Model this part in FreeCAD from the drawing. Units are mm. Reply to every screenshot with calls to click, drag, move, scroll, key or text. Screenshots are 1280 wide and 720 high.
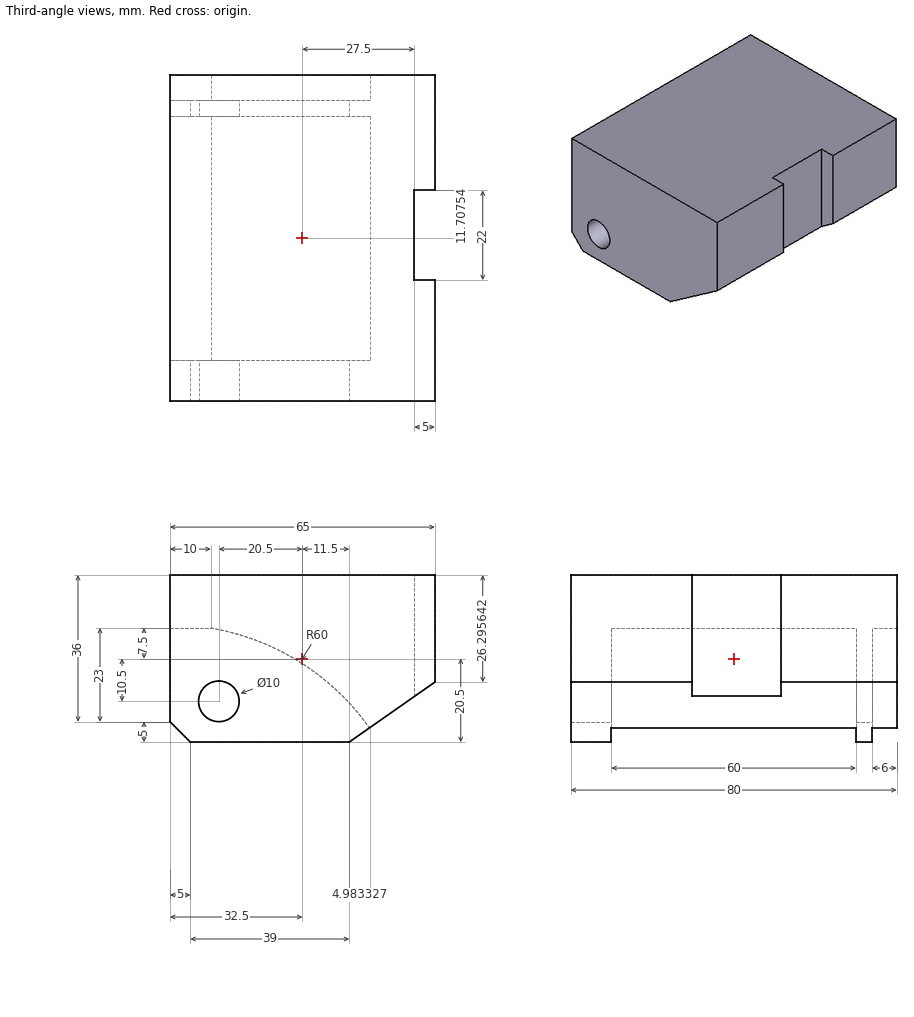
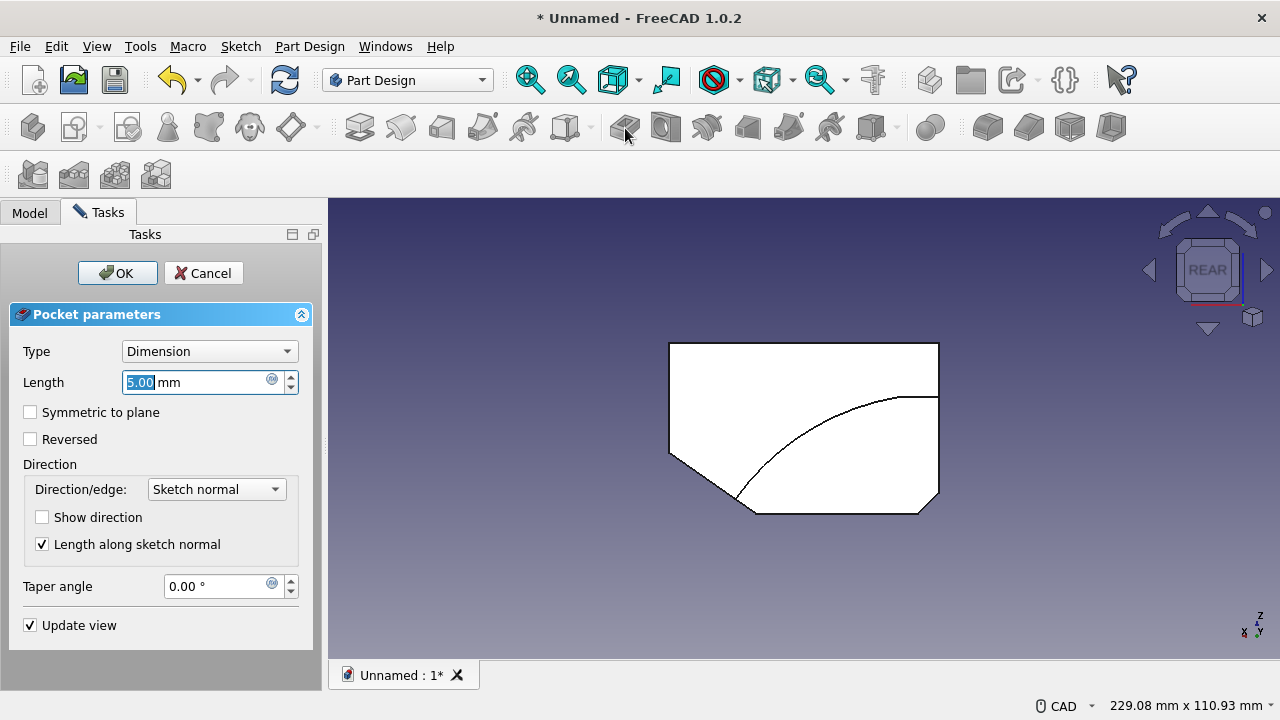
text(60)
key(Tab)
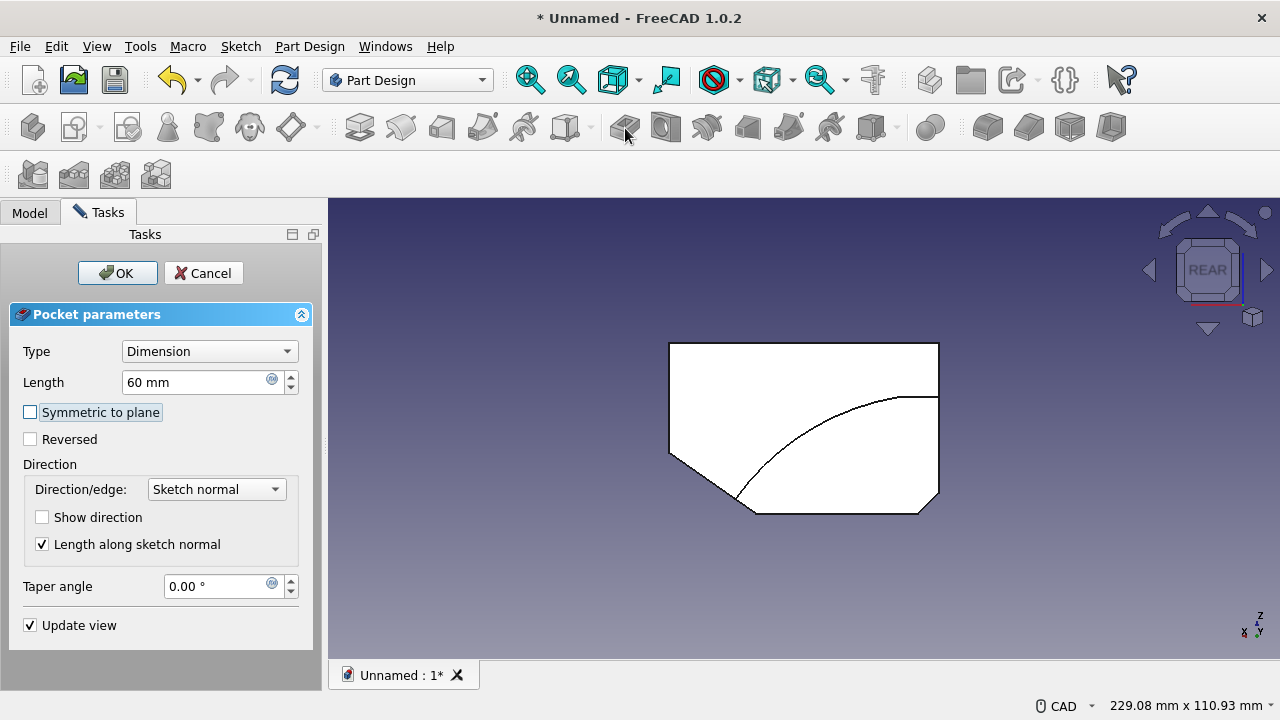
click(31, 412)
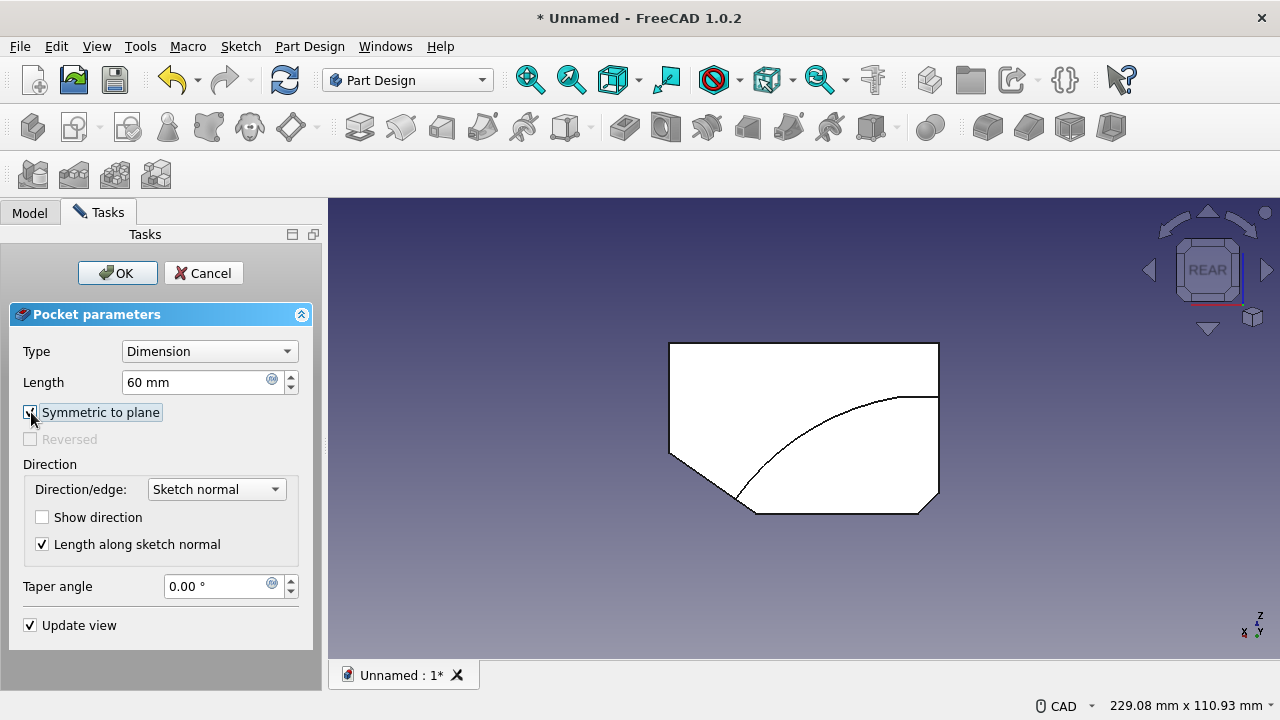
click(118, 273)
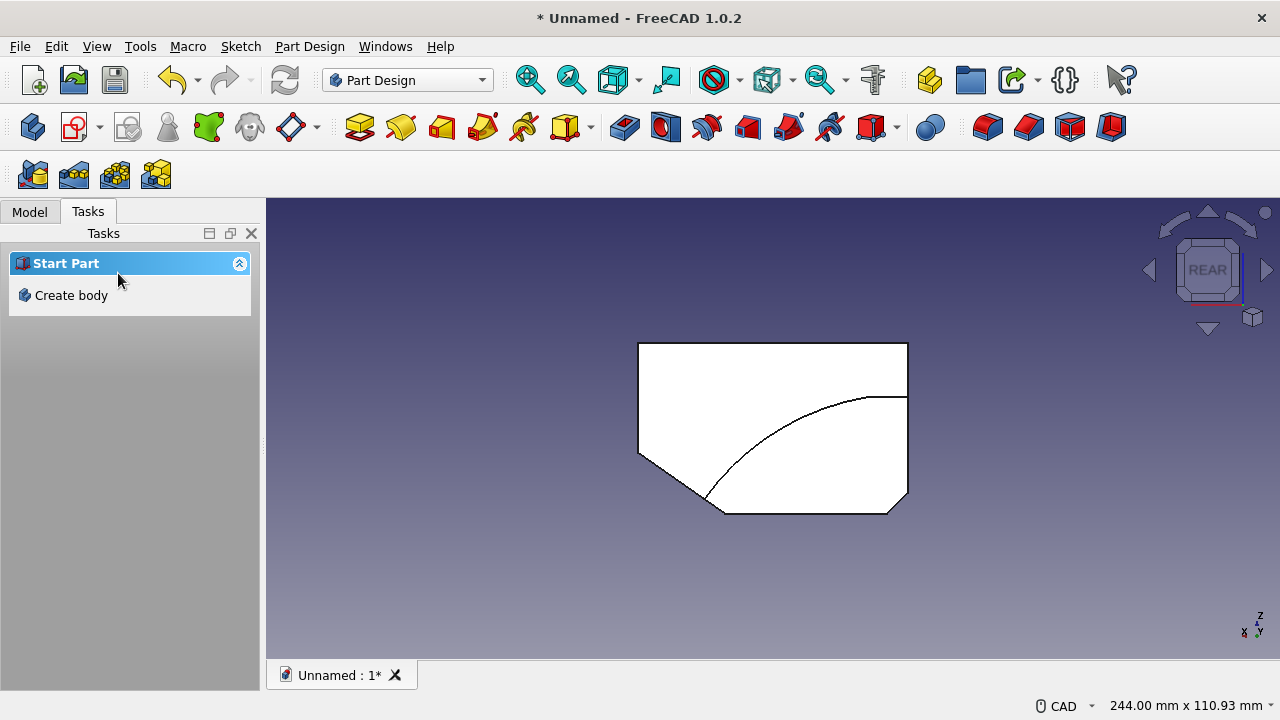
key(v)
key(f)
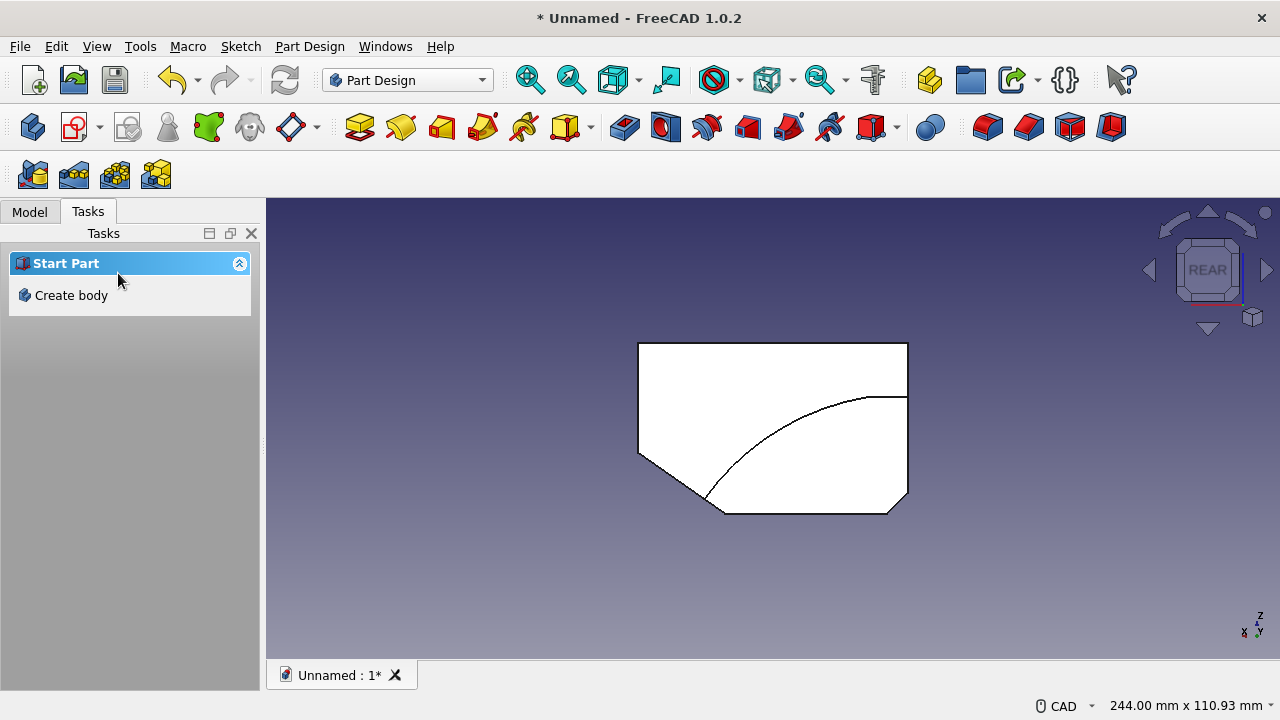
click(835, 455)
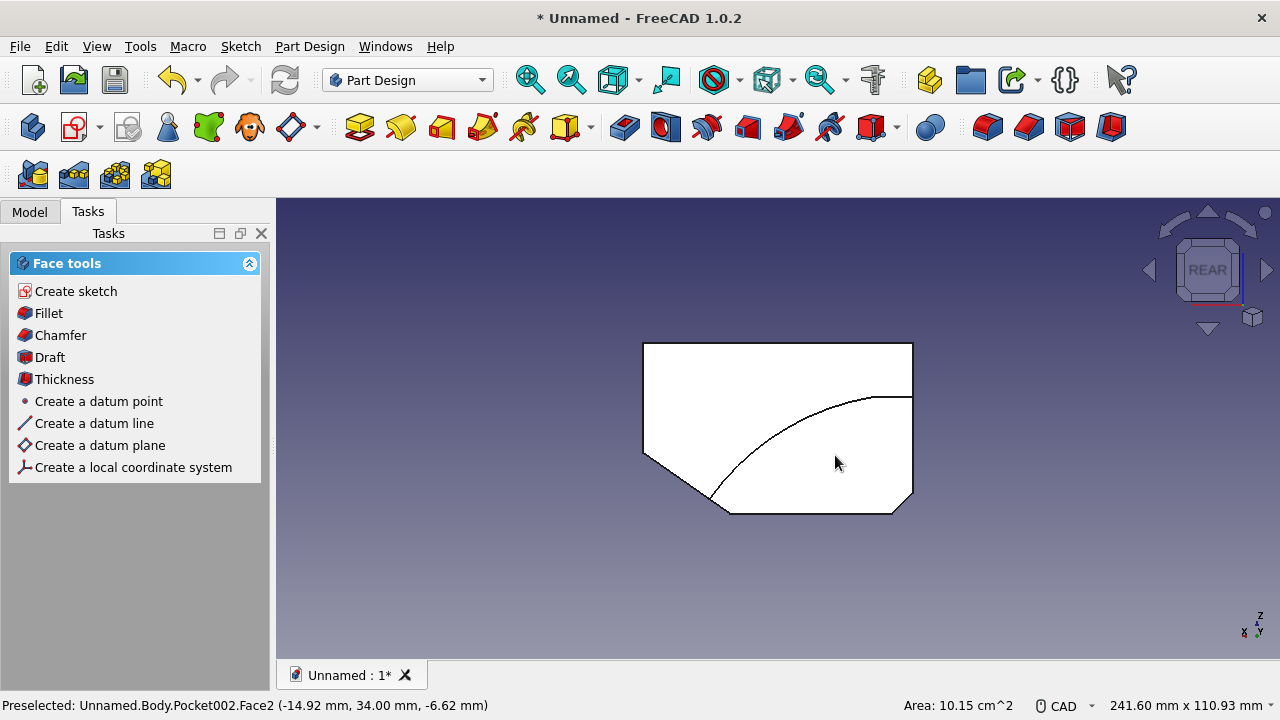
click(74, 128)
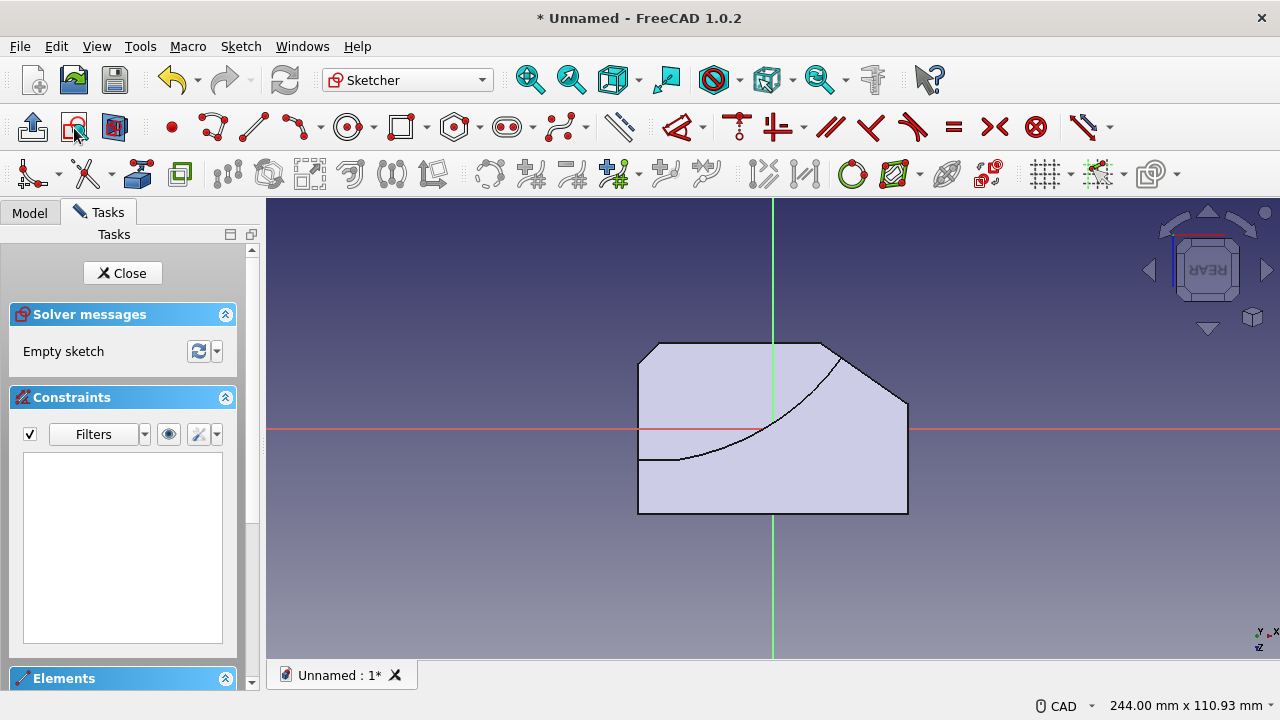
scroll(685, 378, up, 10)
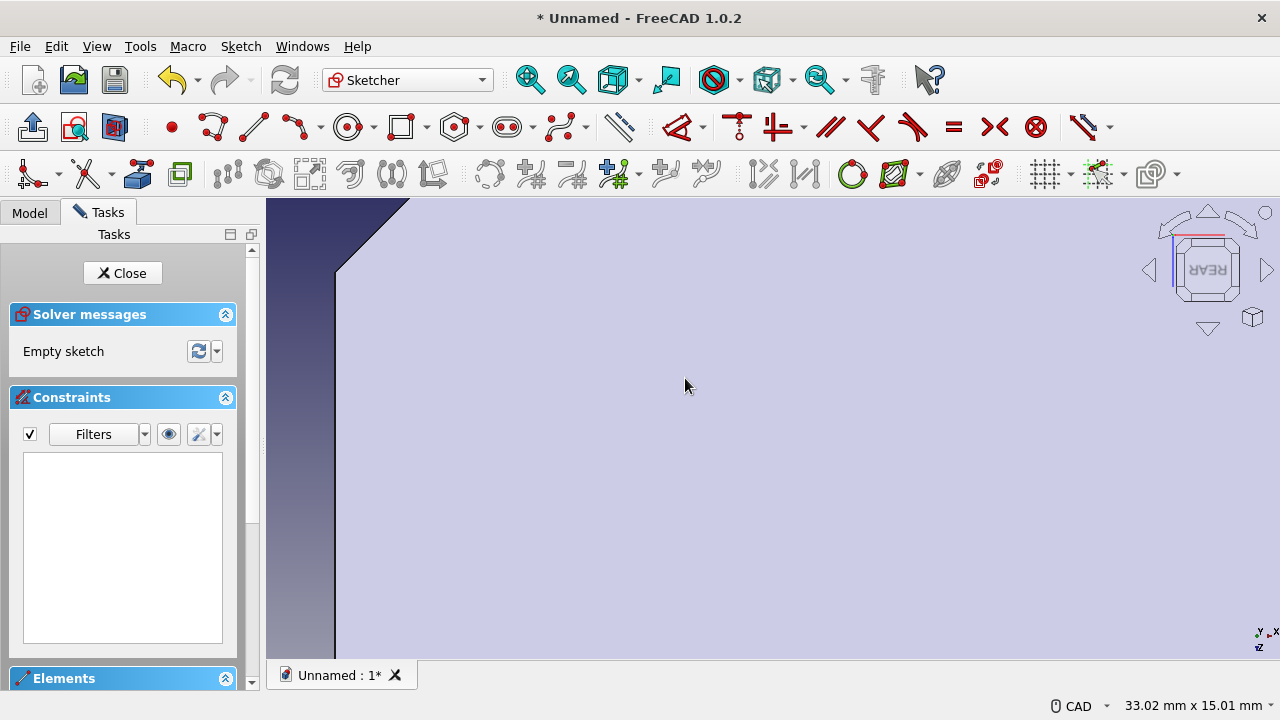
key(g)
key(c)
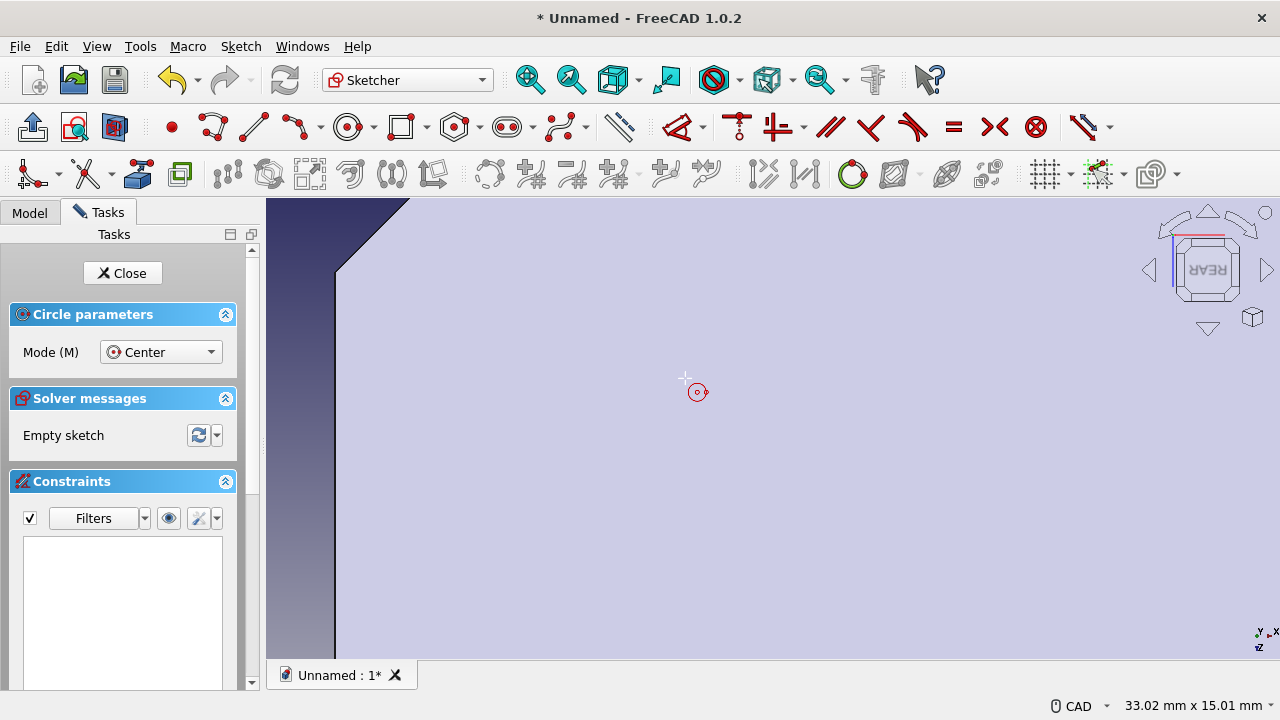
click(703, 426)
click(812, 318)
key(Escape)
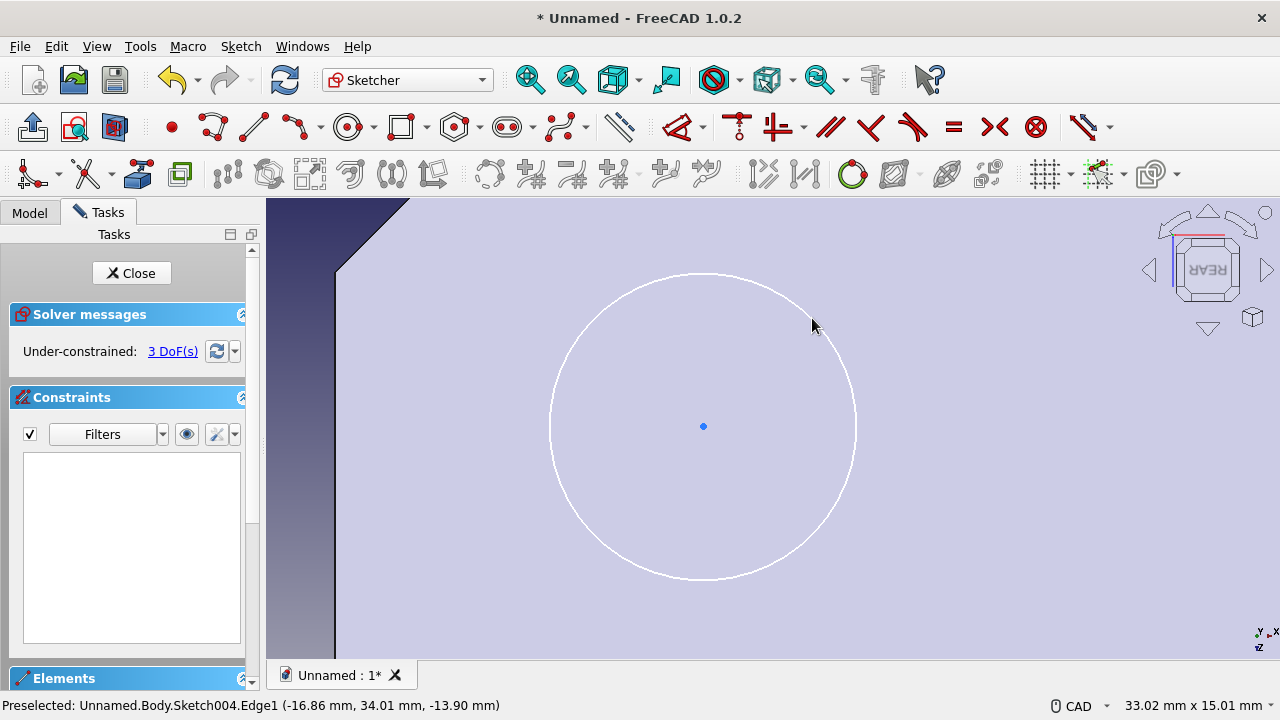
key(d)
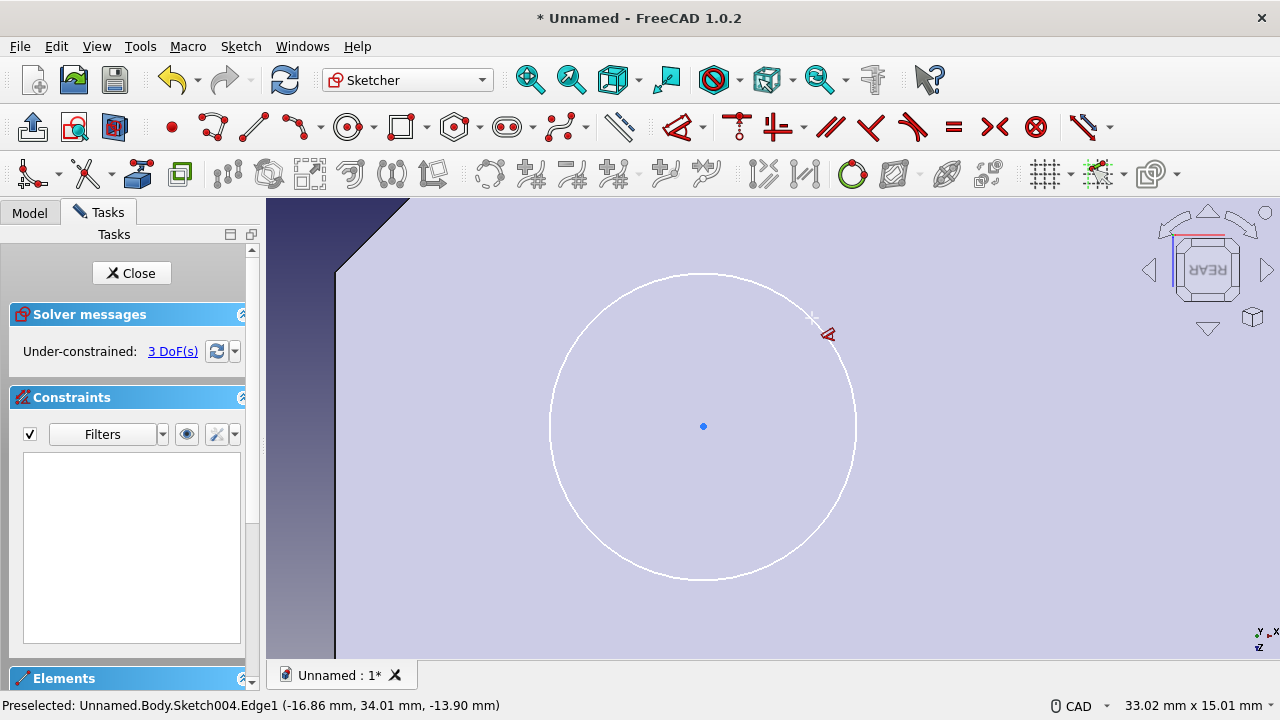
click(811, 318)
click(834, 295)